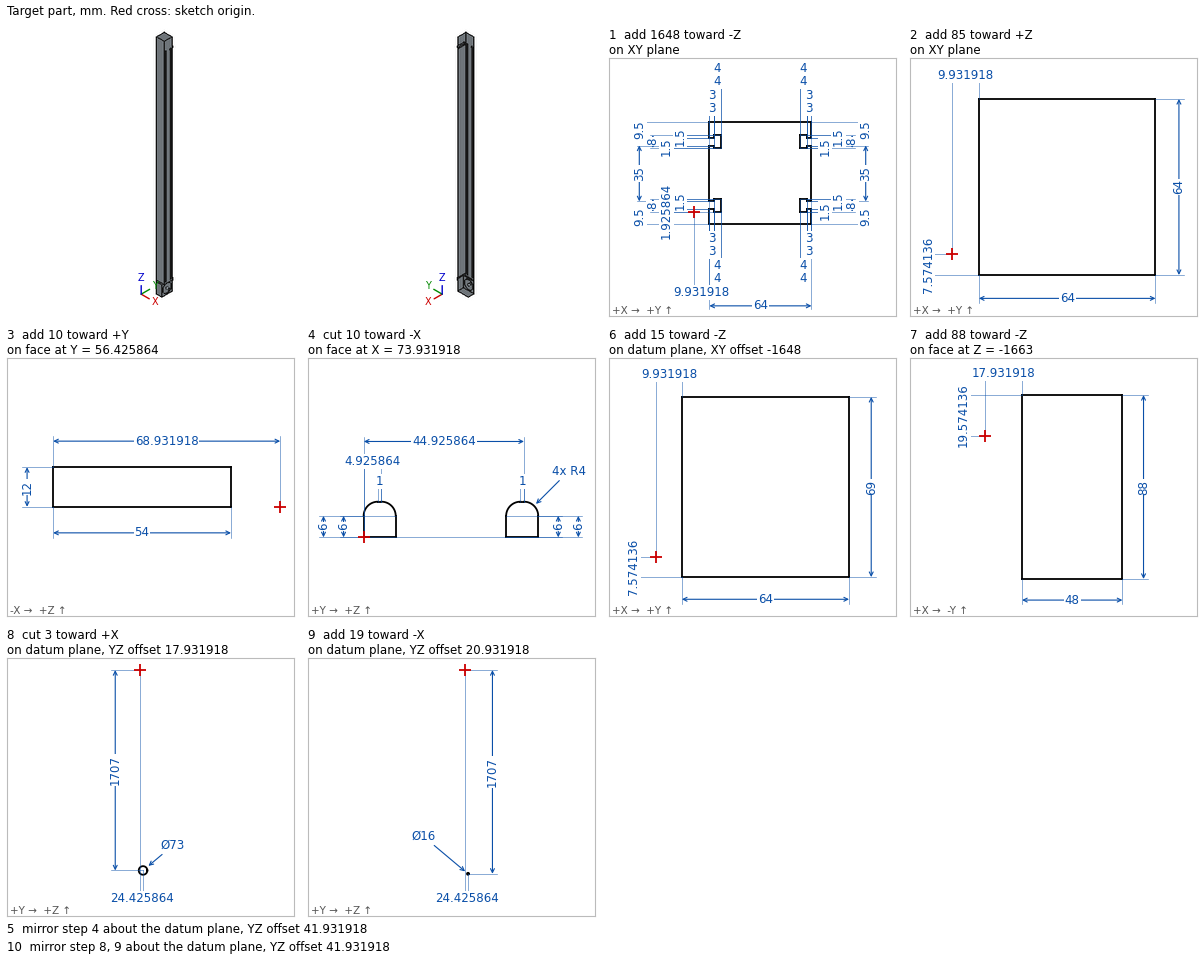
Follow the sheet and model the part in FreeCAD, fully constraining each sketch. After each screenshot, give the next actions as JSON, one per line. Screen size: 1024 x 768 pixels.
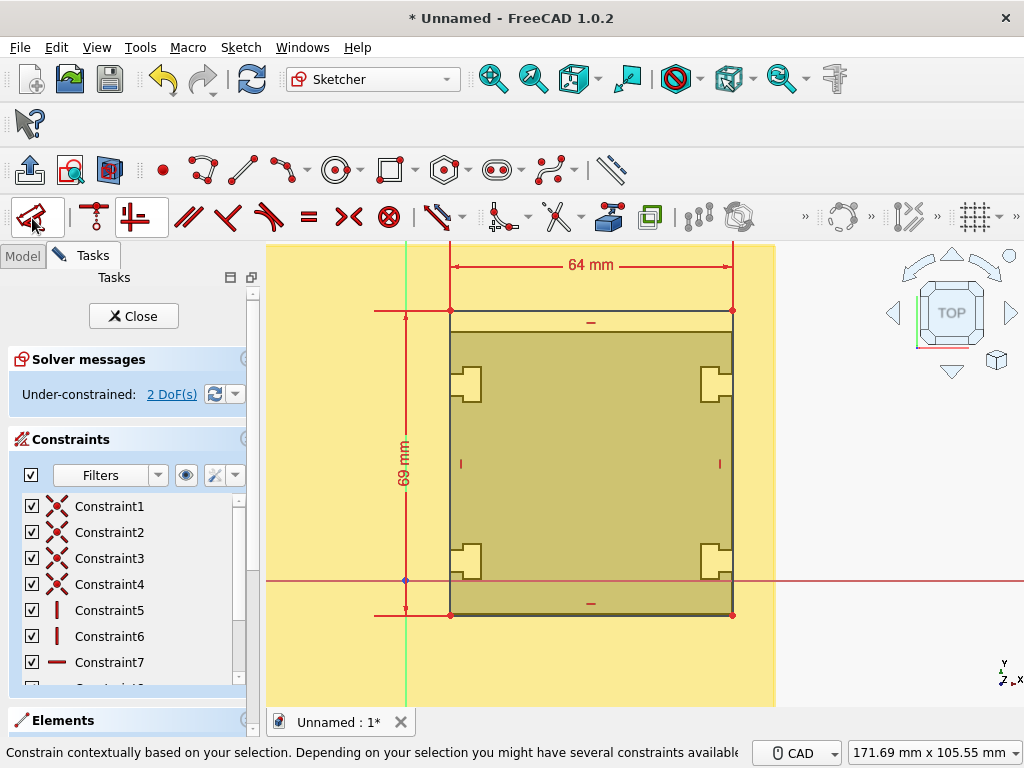
{"action": "left_click", "coordinate": [450, 311]}
{"action": "left_click", "coordinate": [428, 277]}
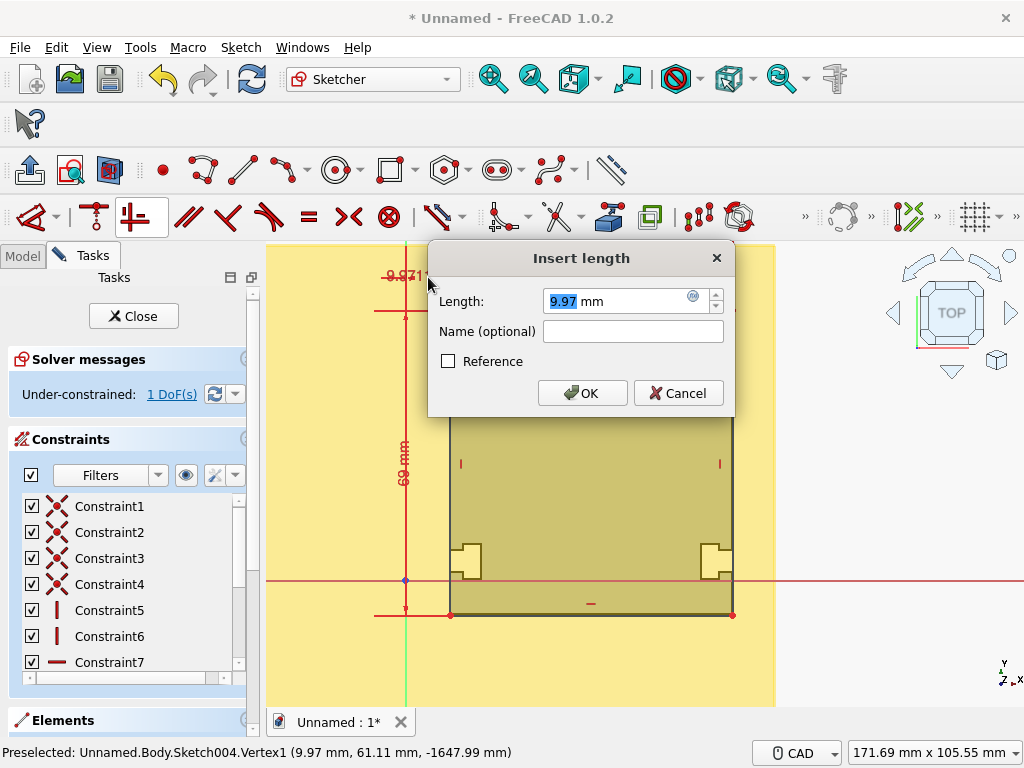
{"action": "type", "text": "9.931918"}
{"action": "key", "text": "Return"}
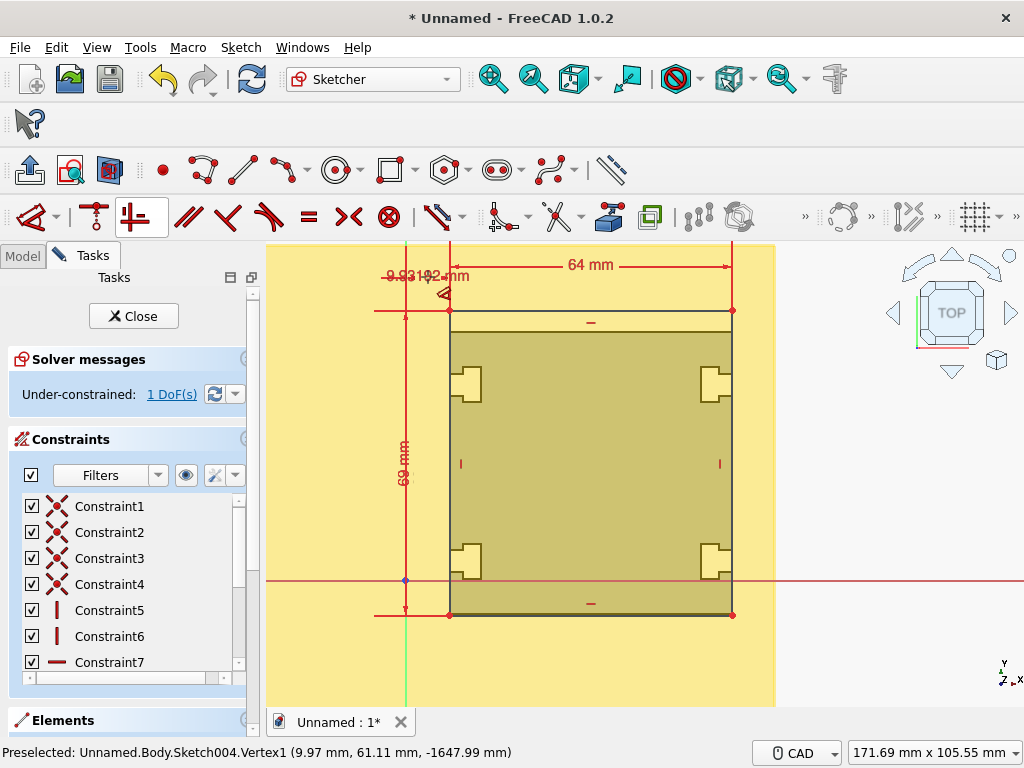
{"action": "left_click", "coordinate": [450, 616]}
{"action": "left_click", "coordinate": [372, 598]}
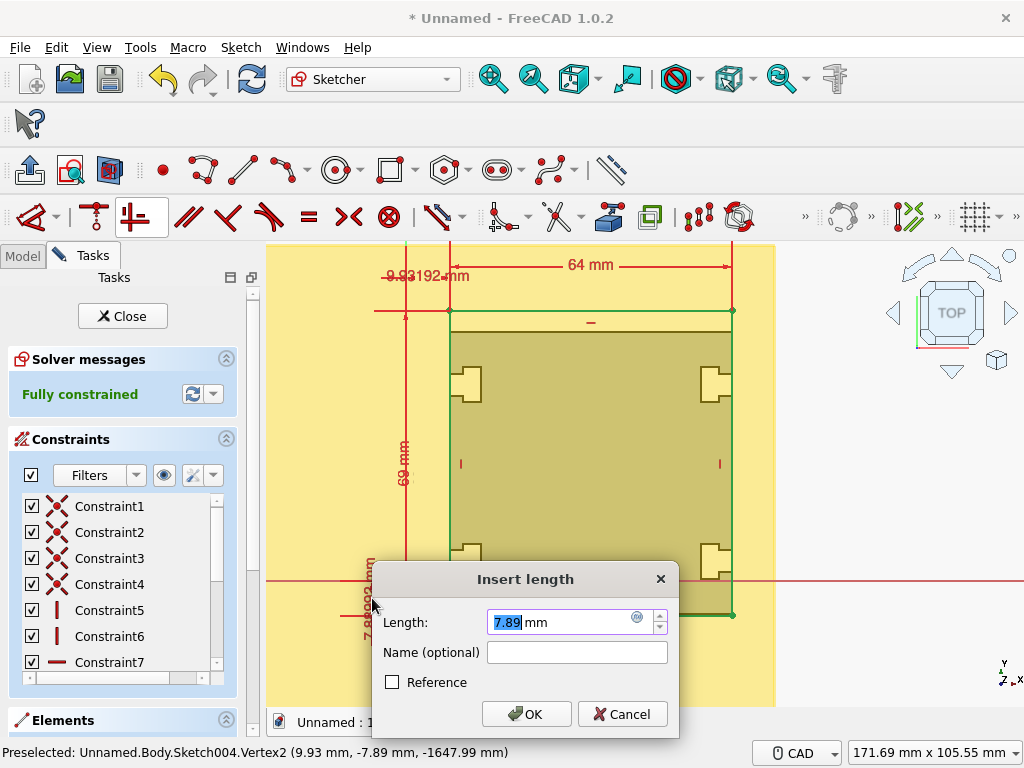
{"action": "type", "text": "7.574136"}
{"action": "key", "text": "Return"}
{"action": "key", "text": "Escape"}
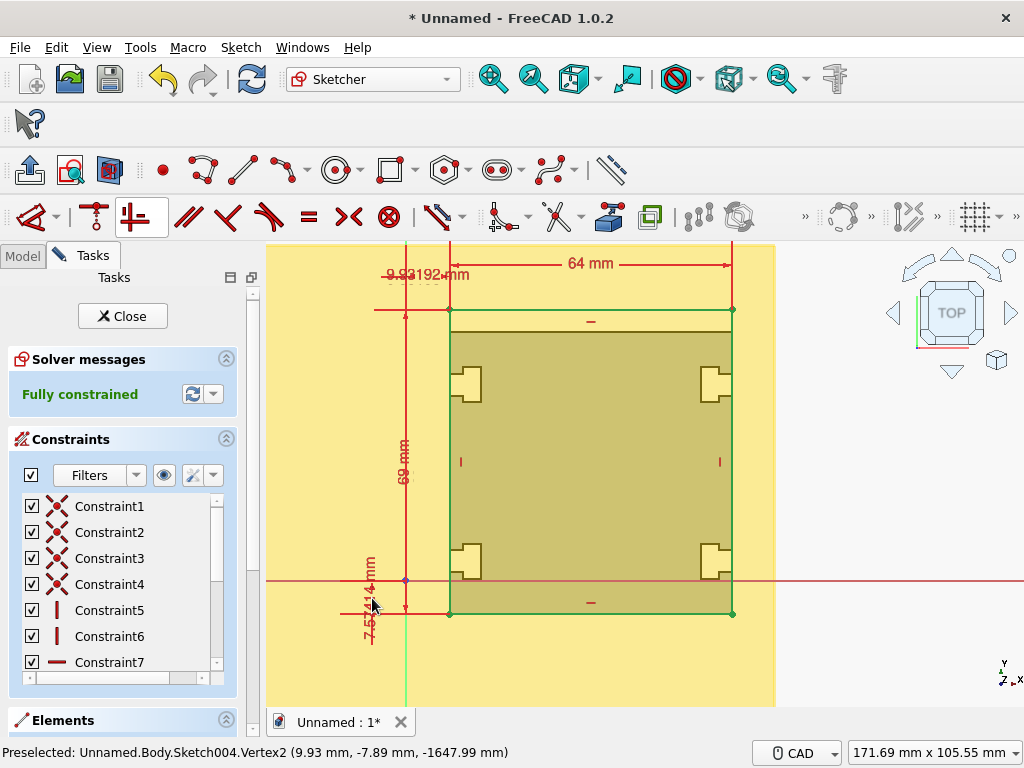
{"action": "left_click", "coordinate": [123, 316]}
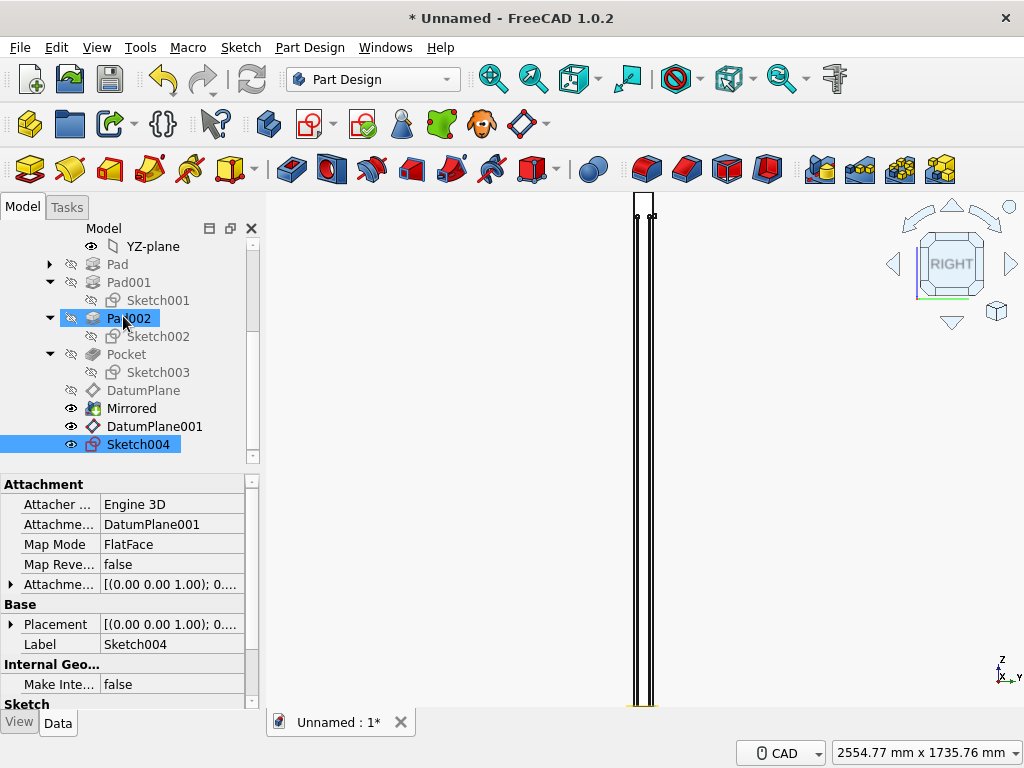
{"action": "left_click", "coordinate": [30, 170]}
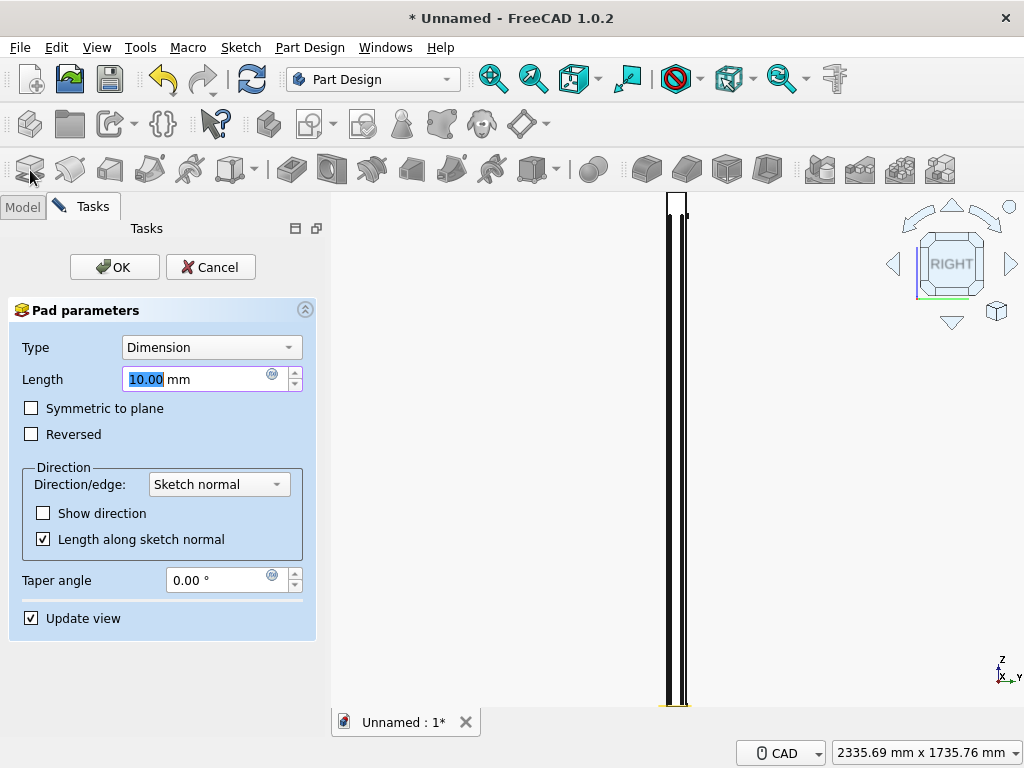
{"action": "type", "text": "15"}
{"action": "key", "text": "Tab"}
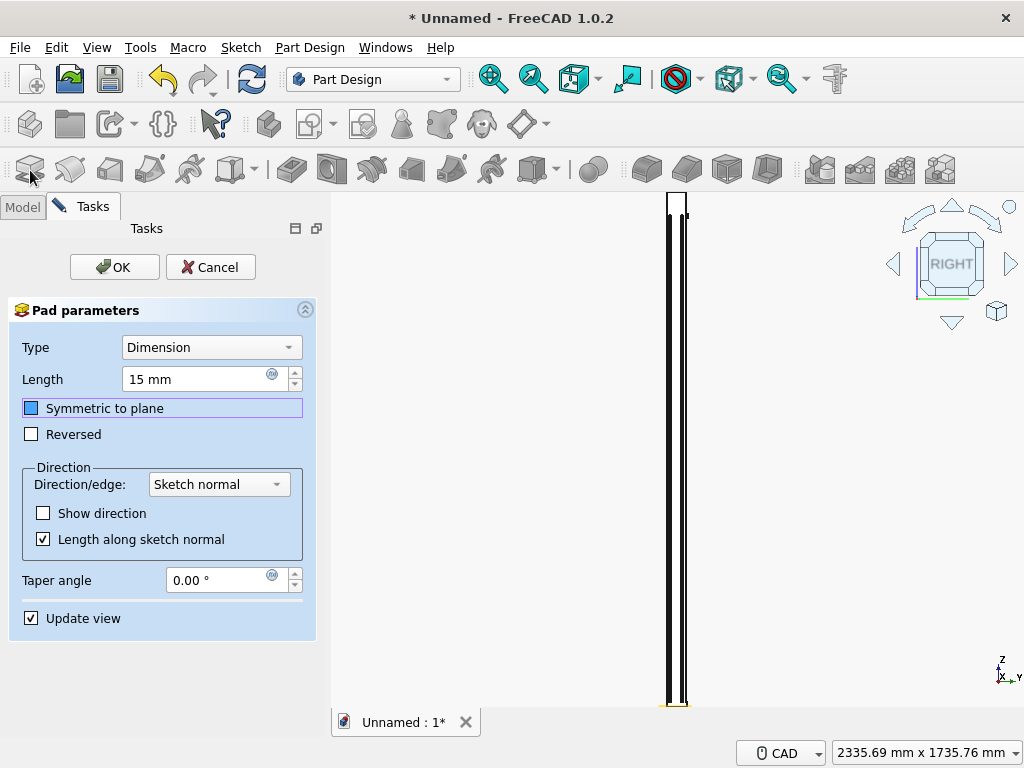
{"action": "left_click", "coordinate": [30, 434]}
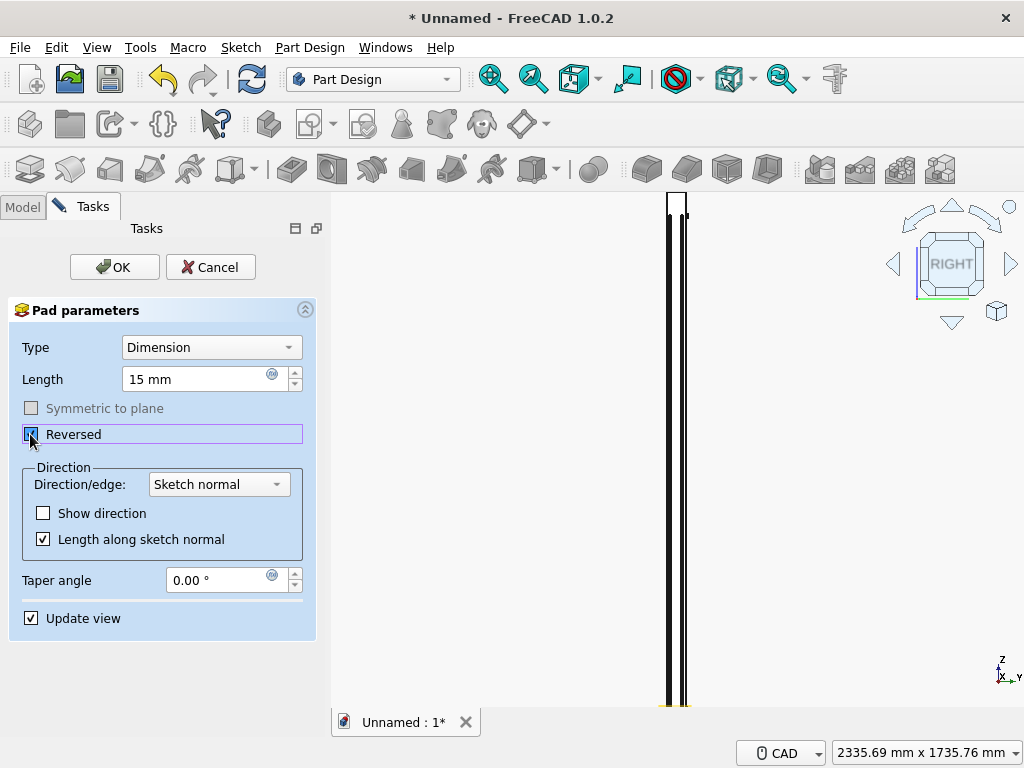
{"action": "left_click", "coordinate": [115, 267]}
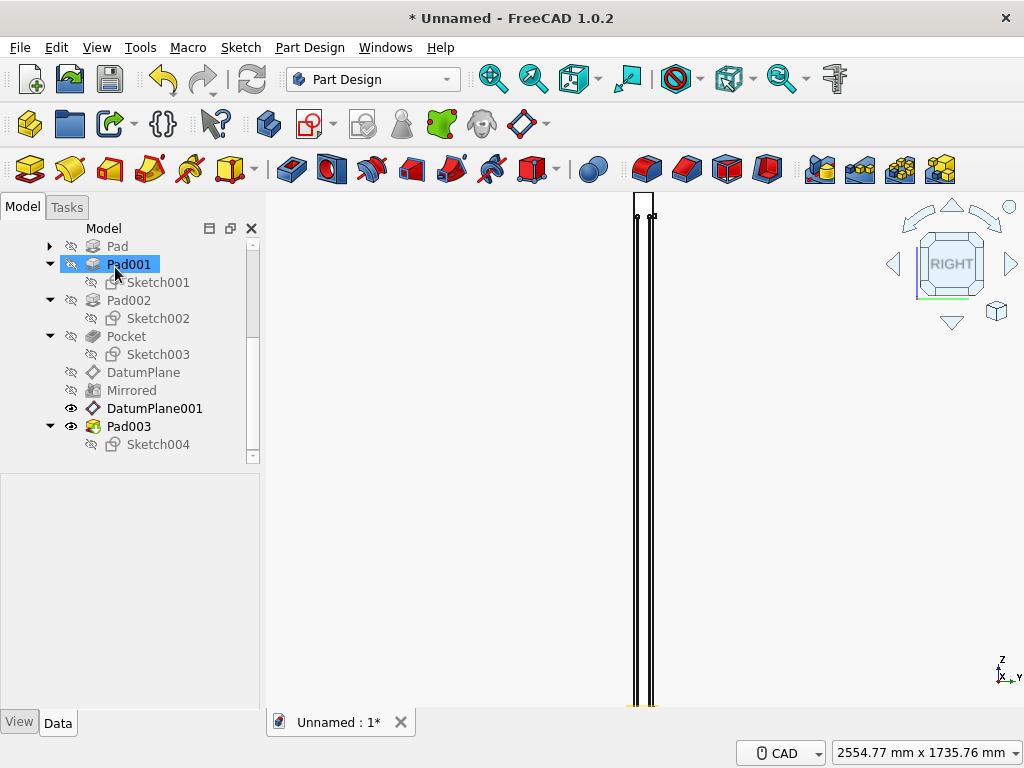
{"action": "left_click", "coordinate": [116, 408]}
{"action": "key", "text": "space"}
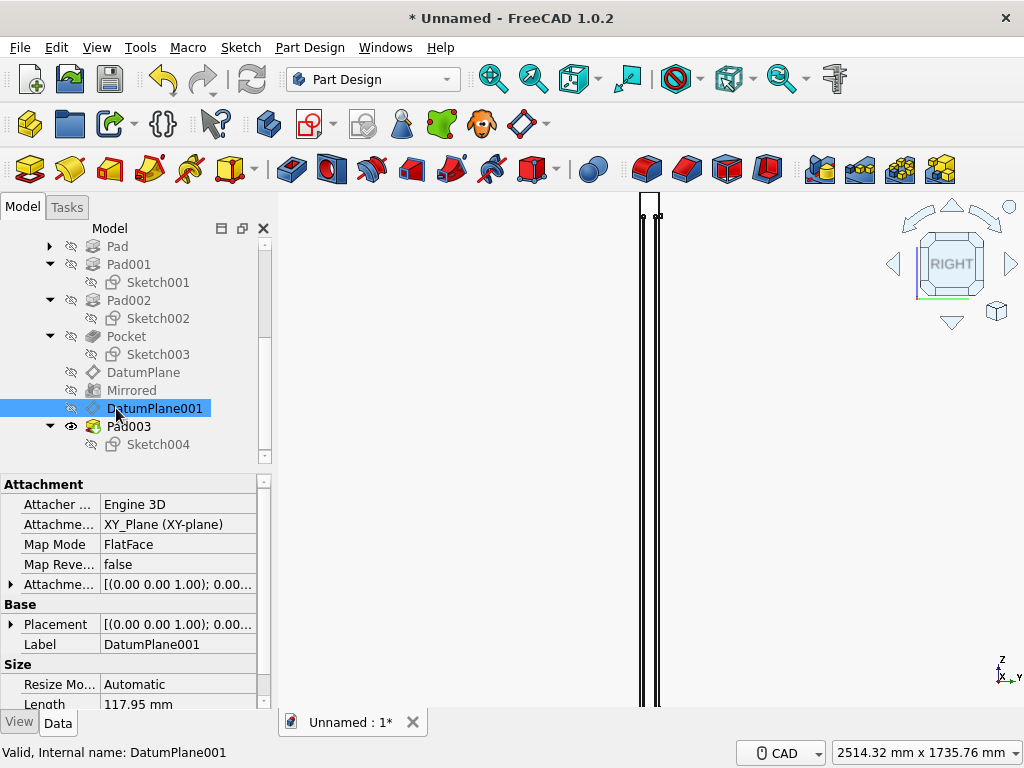
{"action": "left_click", "coordinate": [494, 80]}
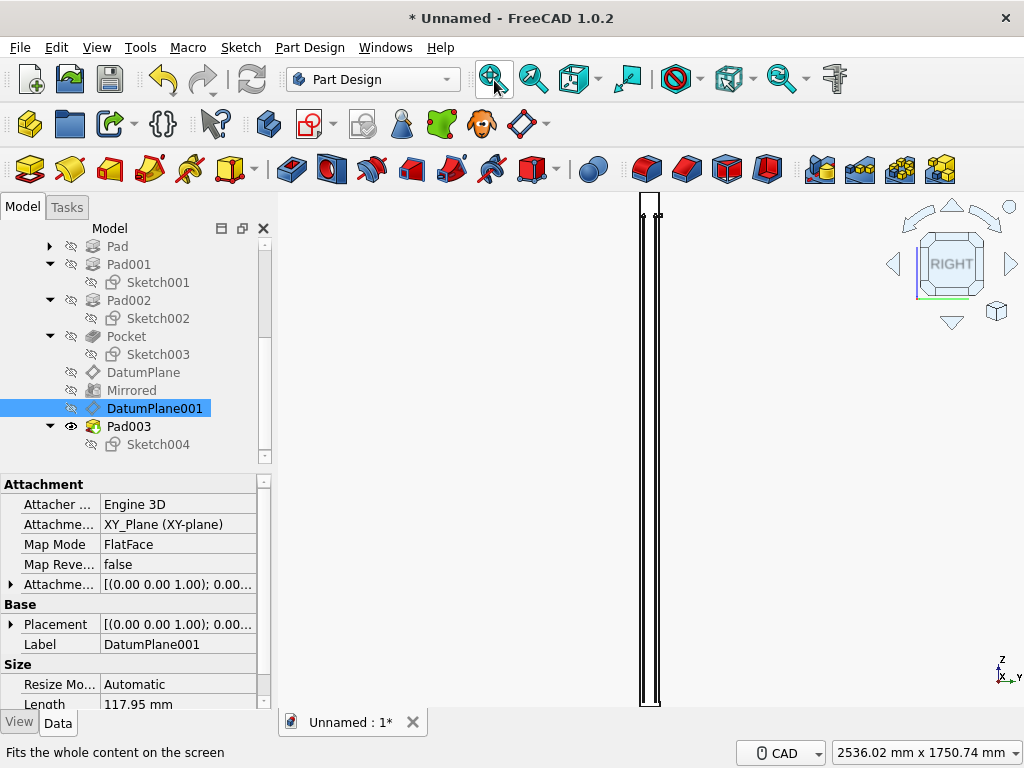
{"action": "key", "text": "5"}